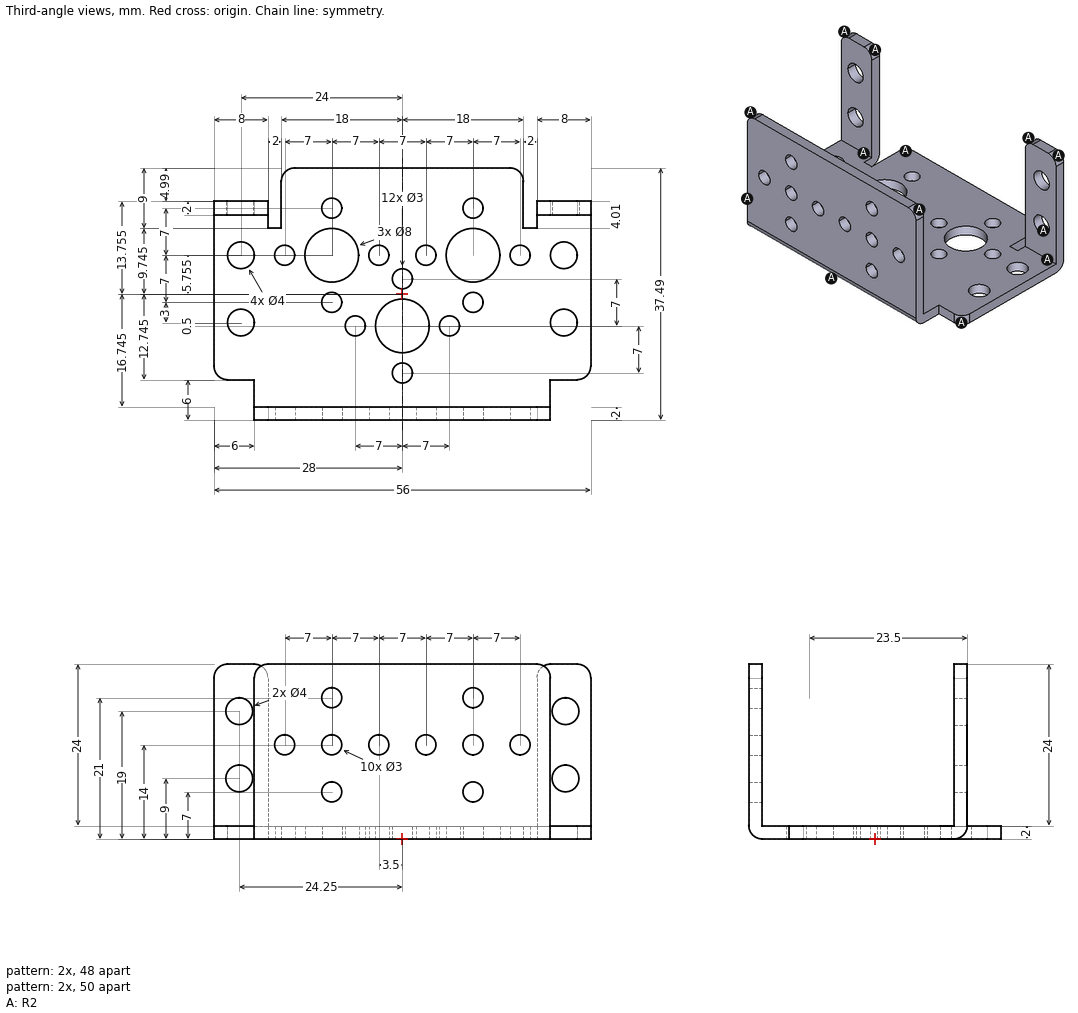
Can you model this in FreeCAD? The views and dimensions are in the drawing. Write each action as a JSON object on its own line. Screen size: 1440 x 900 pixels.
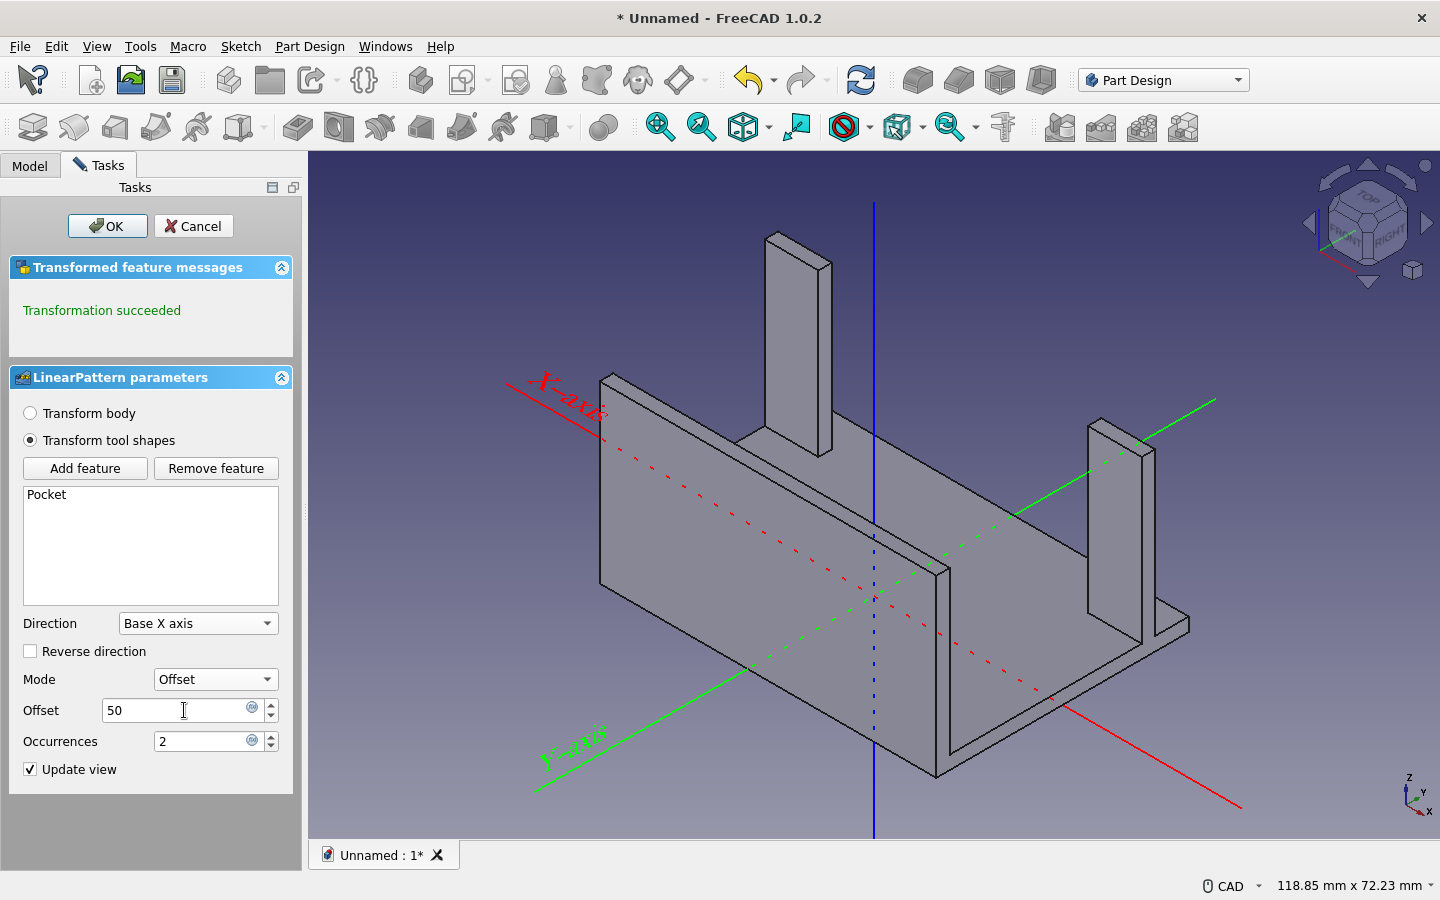
{"action": "triple_click", "coordinate": [210, 742]}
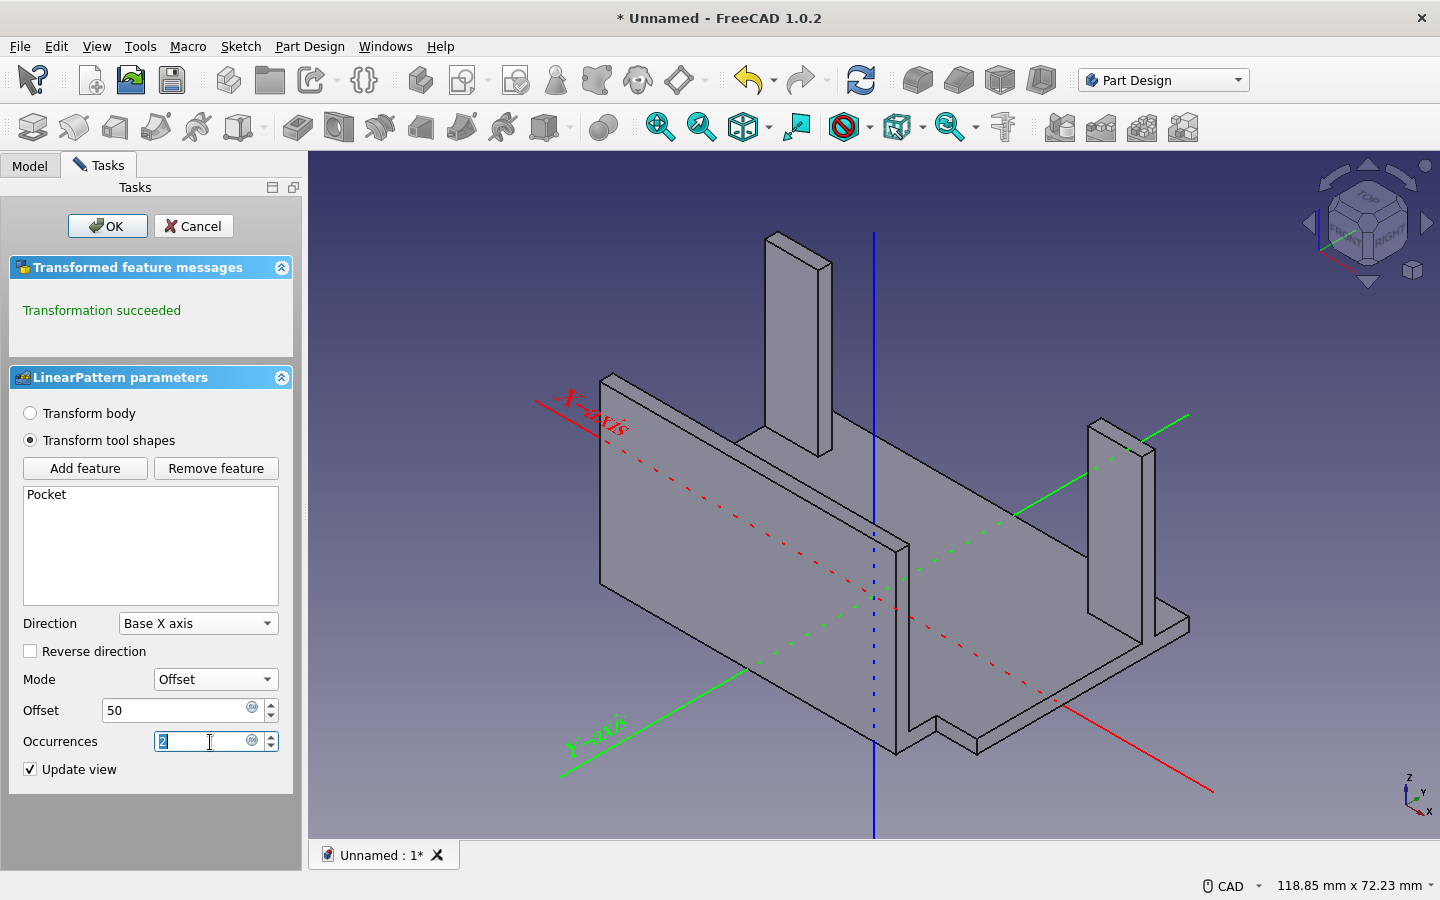
{"action": "type", "text": "2"}
{"action": "key", "text": "Tab"}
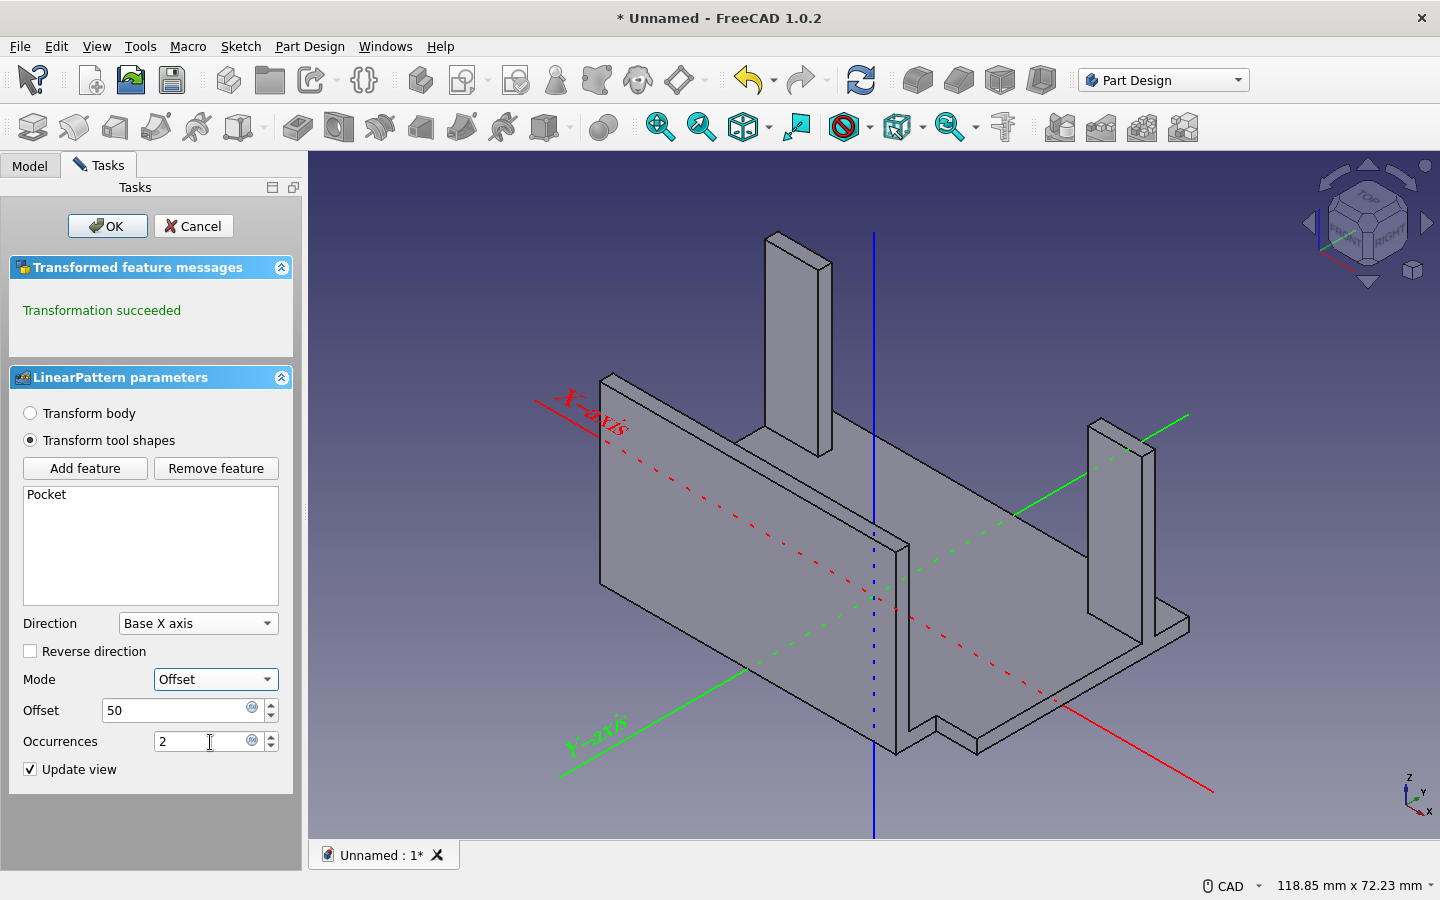
{"action": "left_click", "coordinate": [108, 226]}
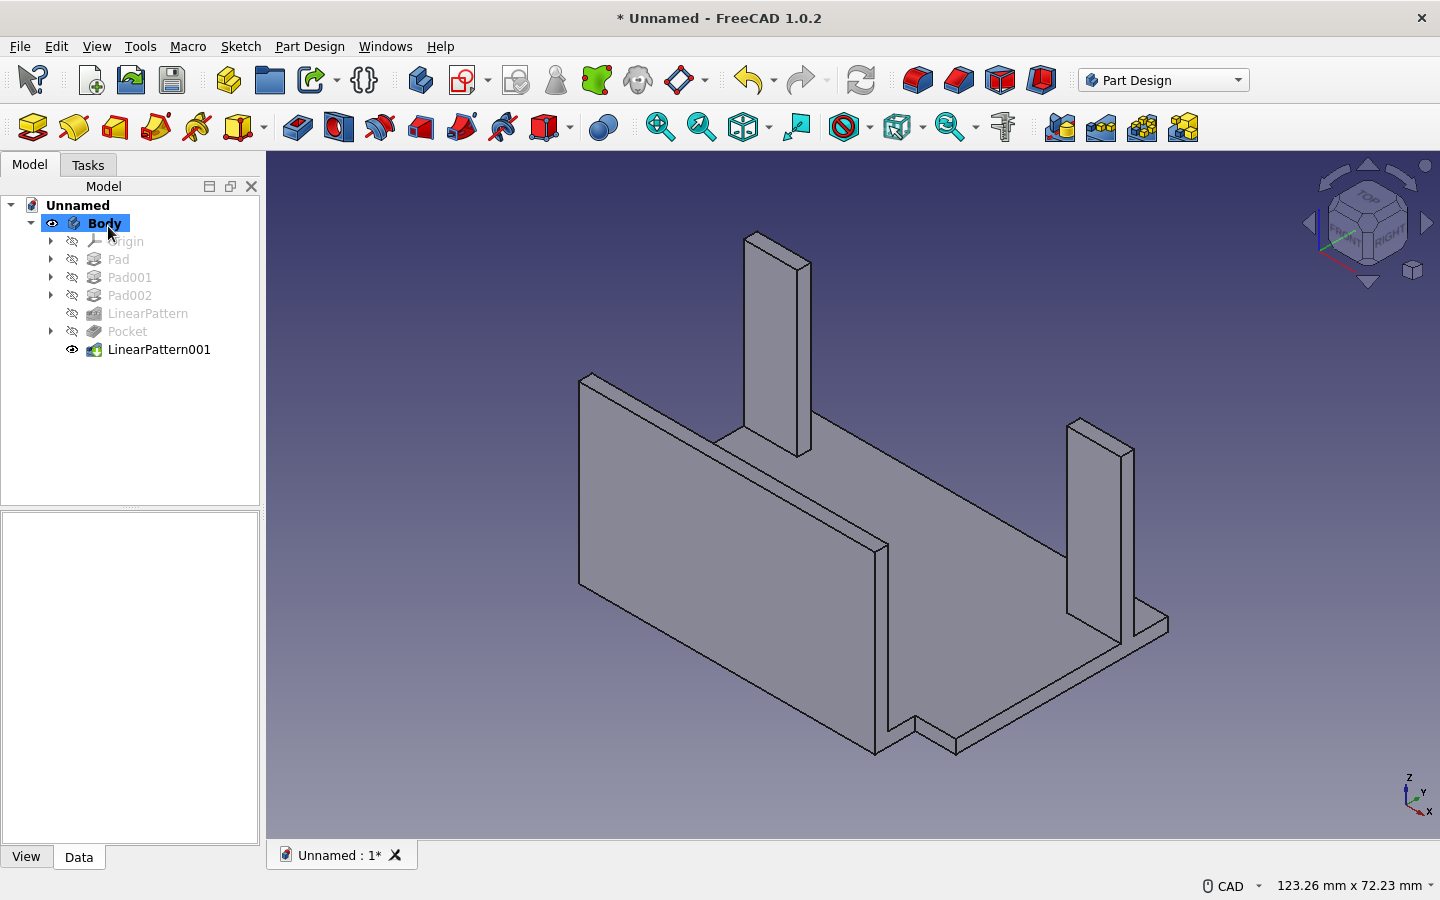
{"action": "left_click", "coordinate": [914, 607]}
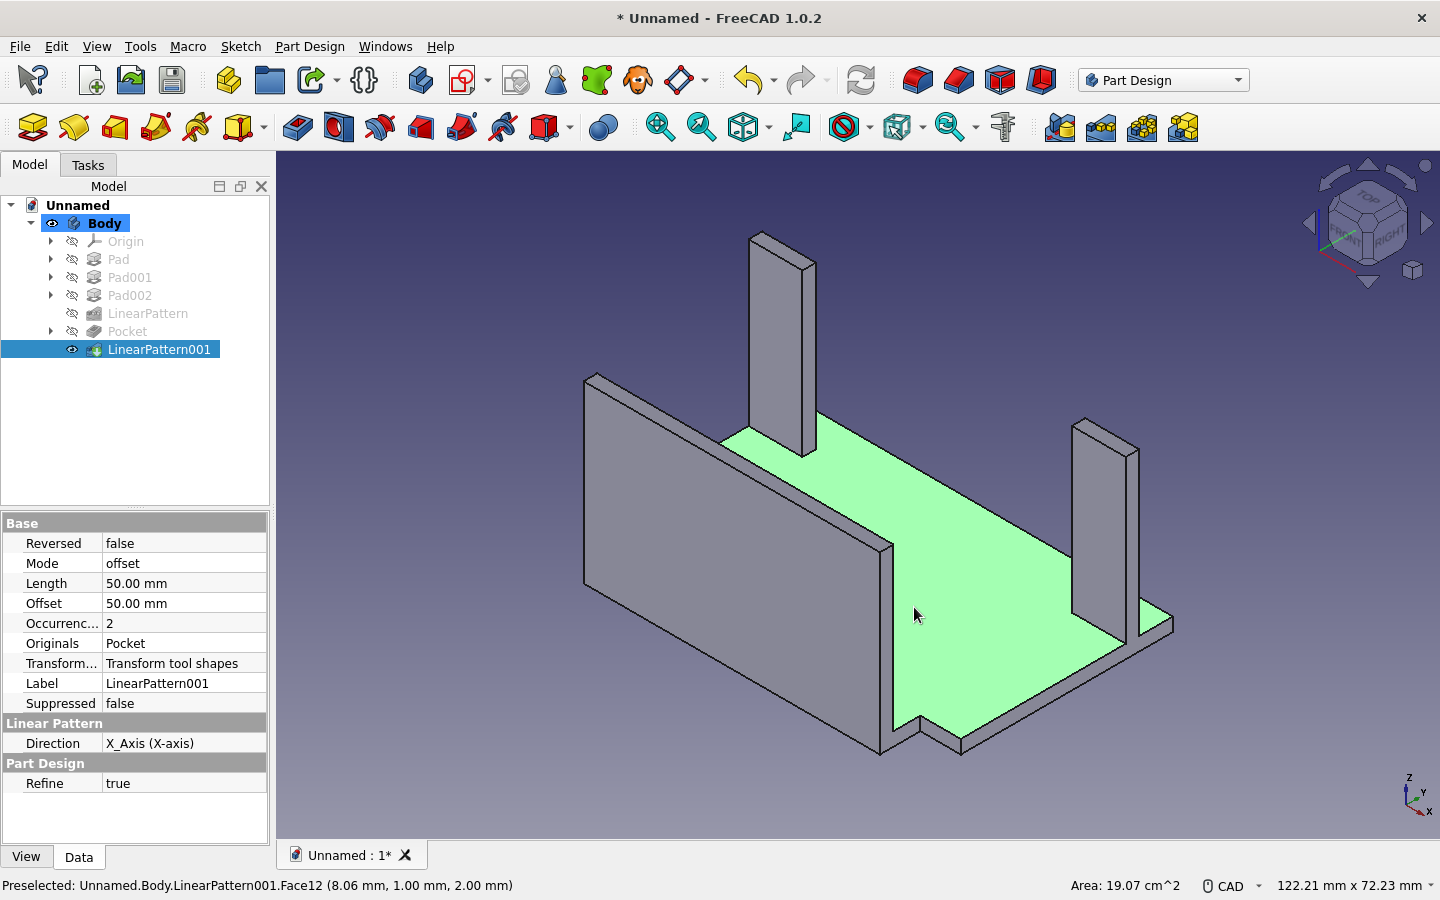
{"action": "left_click", "coordinate": [462, 80]}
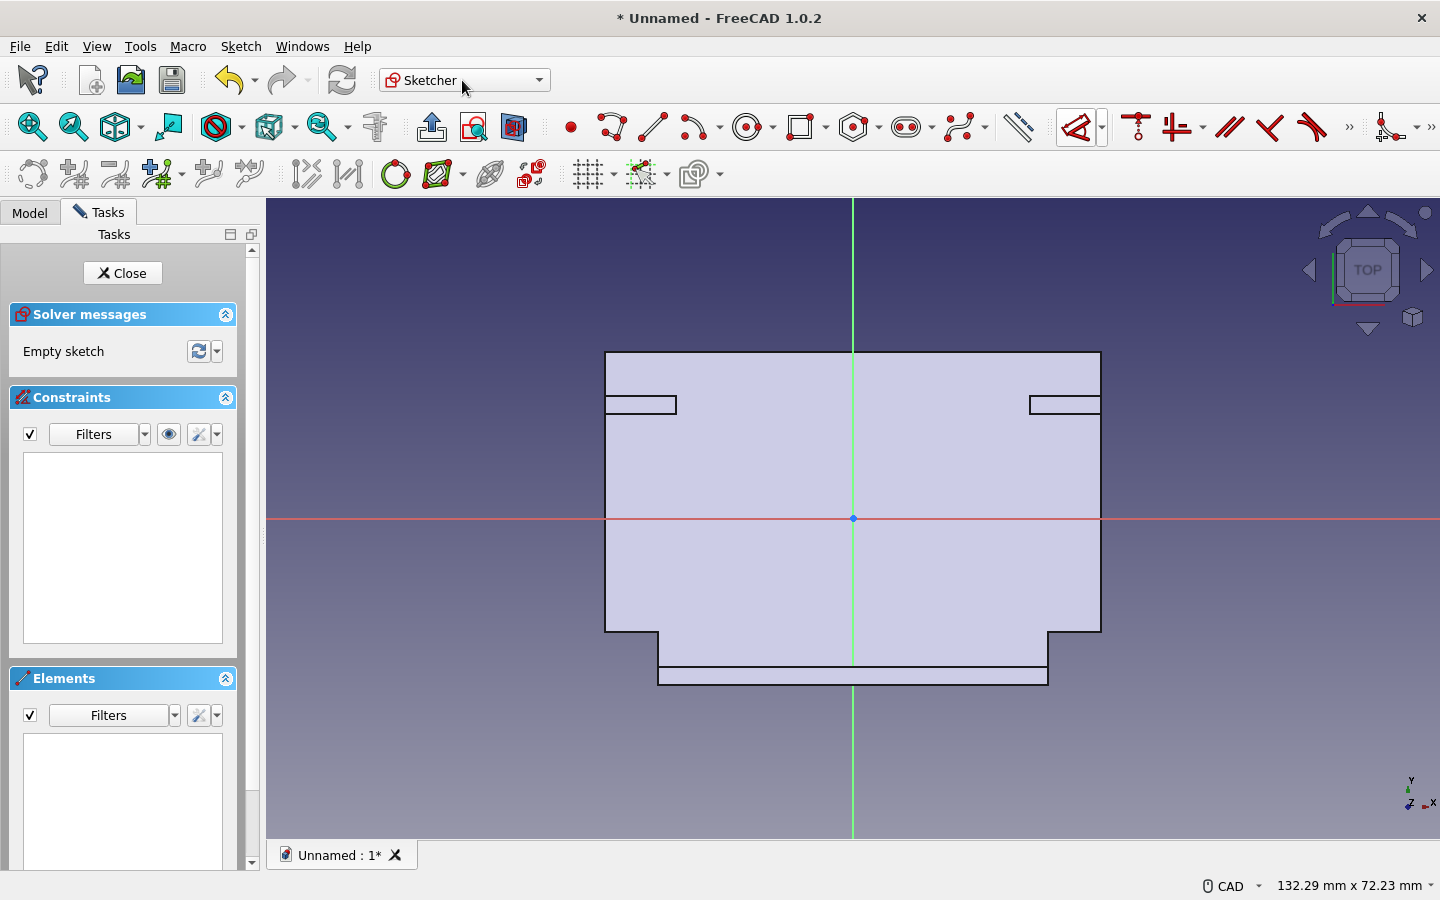
{"action": "scroll", "coordinate": [615, 360], "scroll_direction": "up", "scroll_amount": 8}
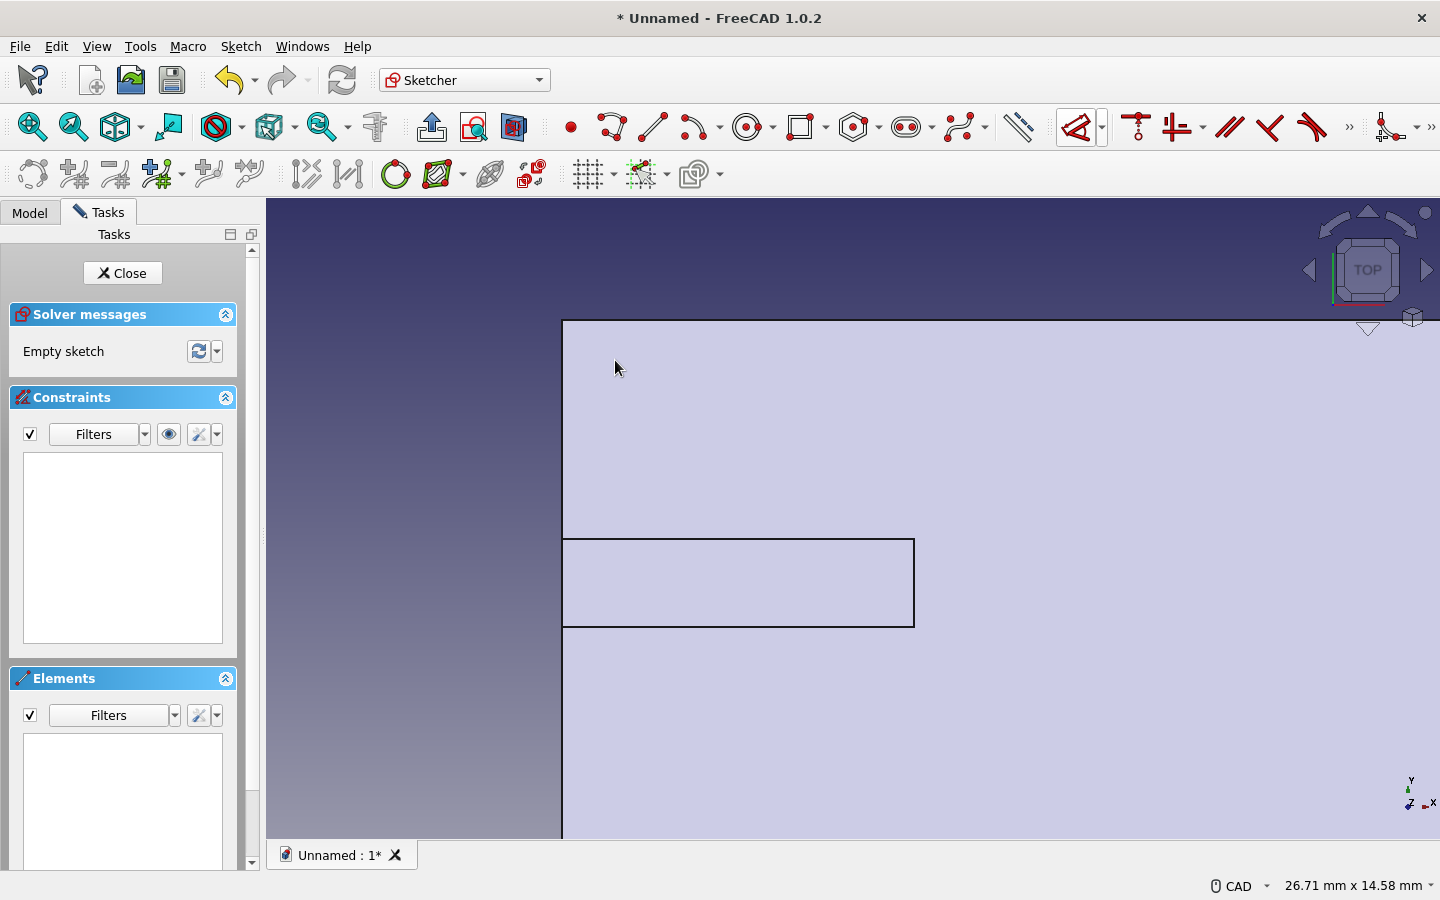
{"action": "key", "text": "g m"}